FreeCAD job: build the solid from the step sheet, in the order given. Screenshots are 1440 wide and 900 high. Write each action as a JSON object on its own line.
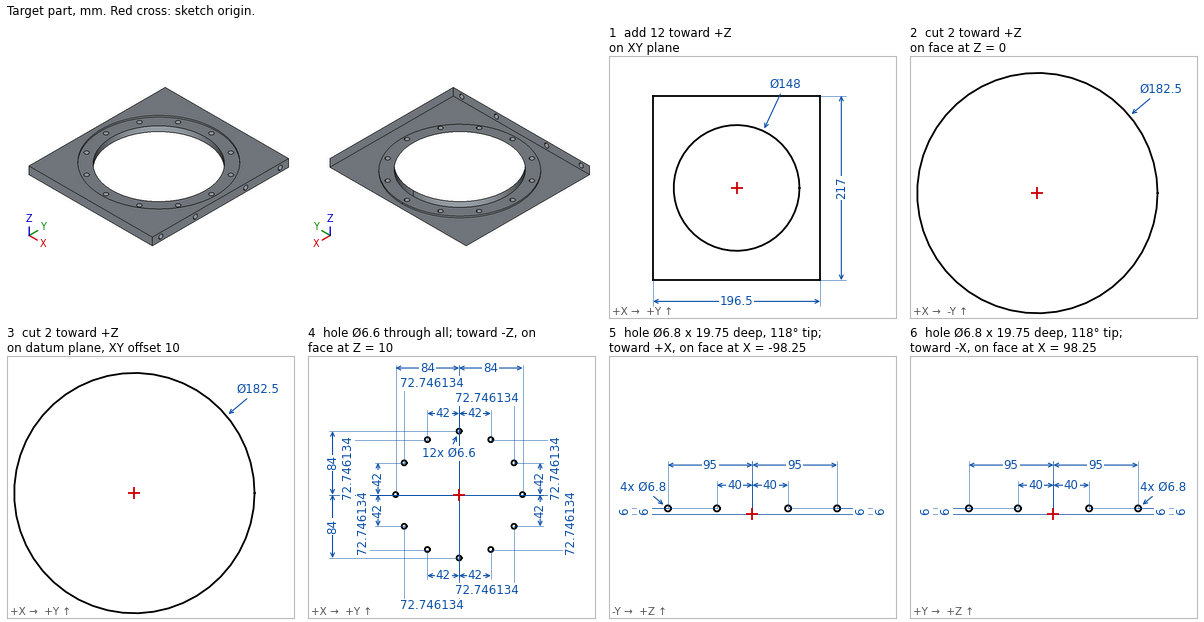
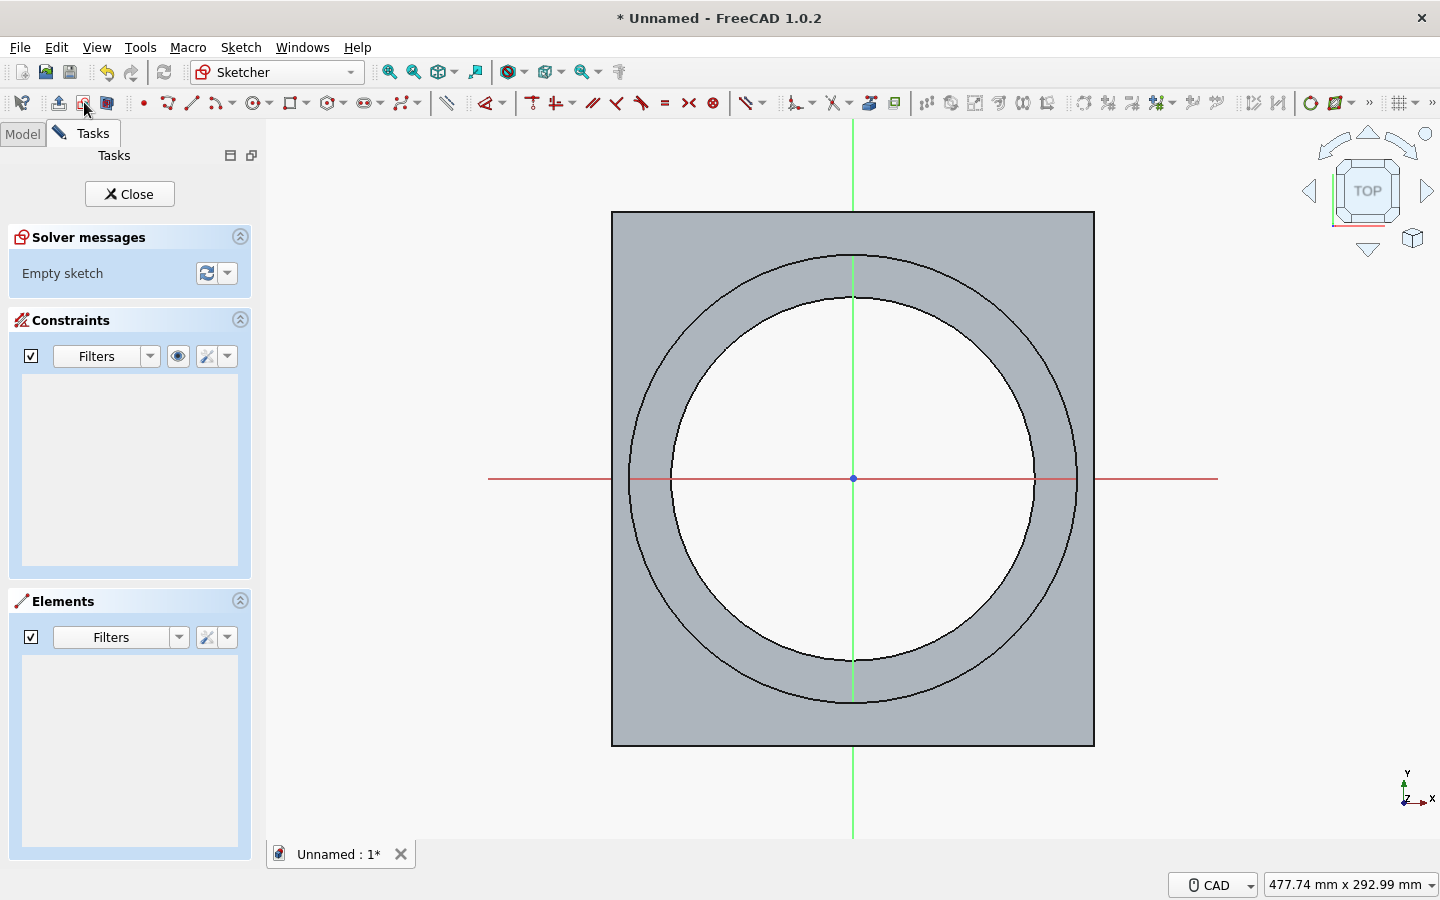
{"action": "left_click", "coordinate": [254, 104]}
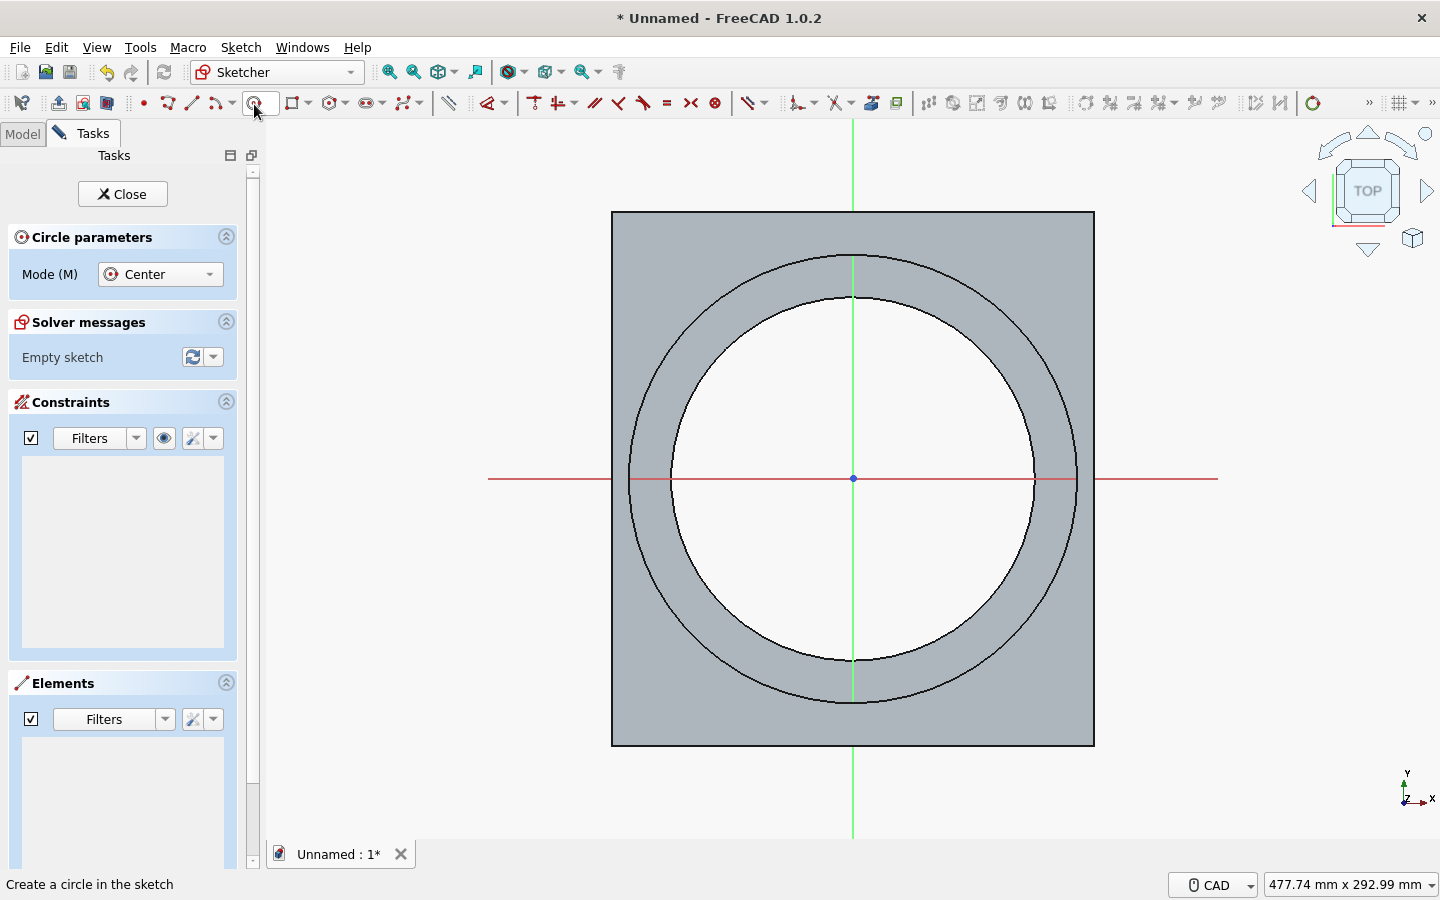
{"action": "scroll", "coordinate": [853, 273], "scroll_direction": "up", "scroll_amount": 6}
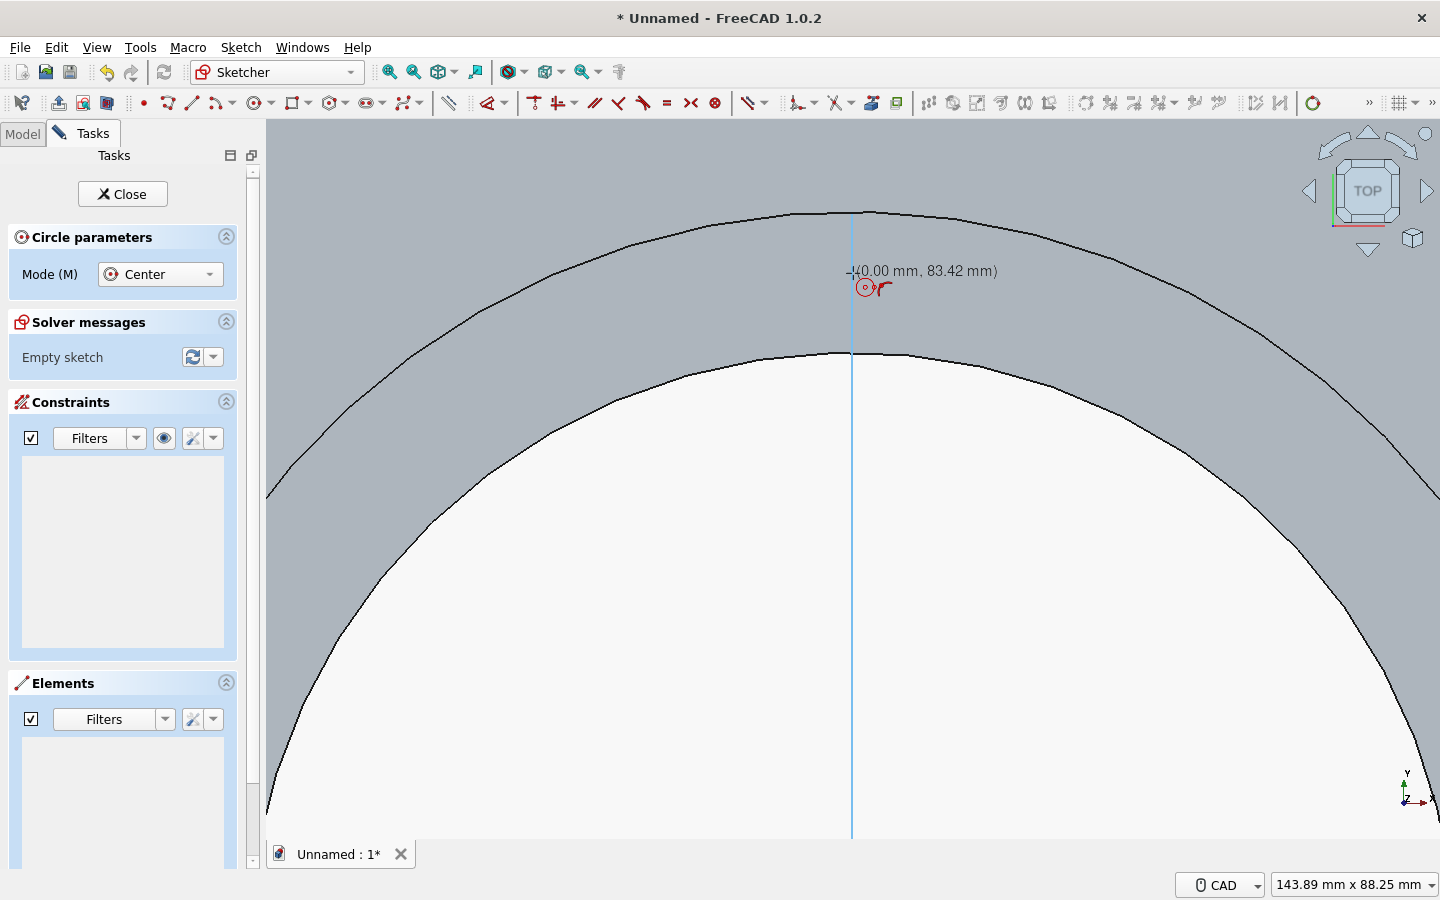
{"action": "left_click", "coordinate": [852, 271]}
{"action": "mouse_move", "coordinate": [871, 252]}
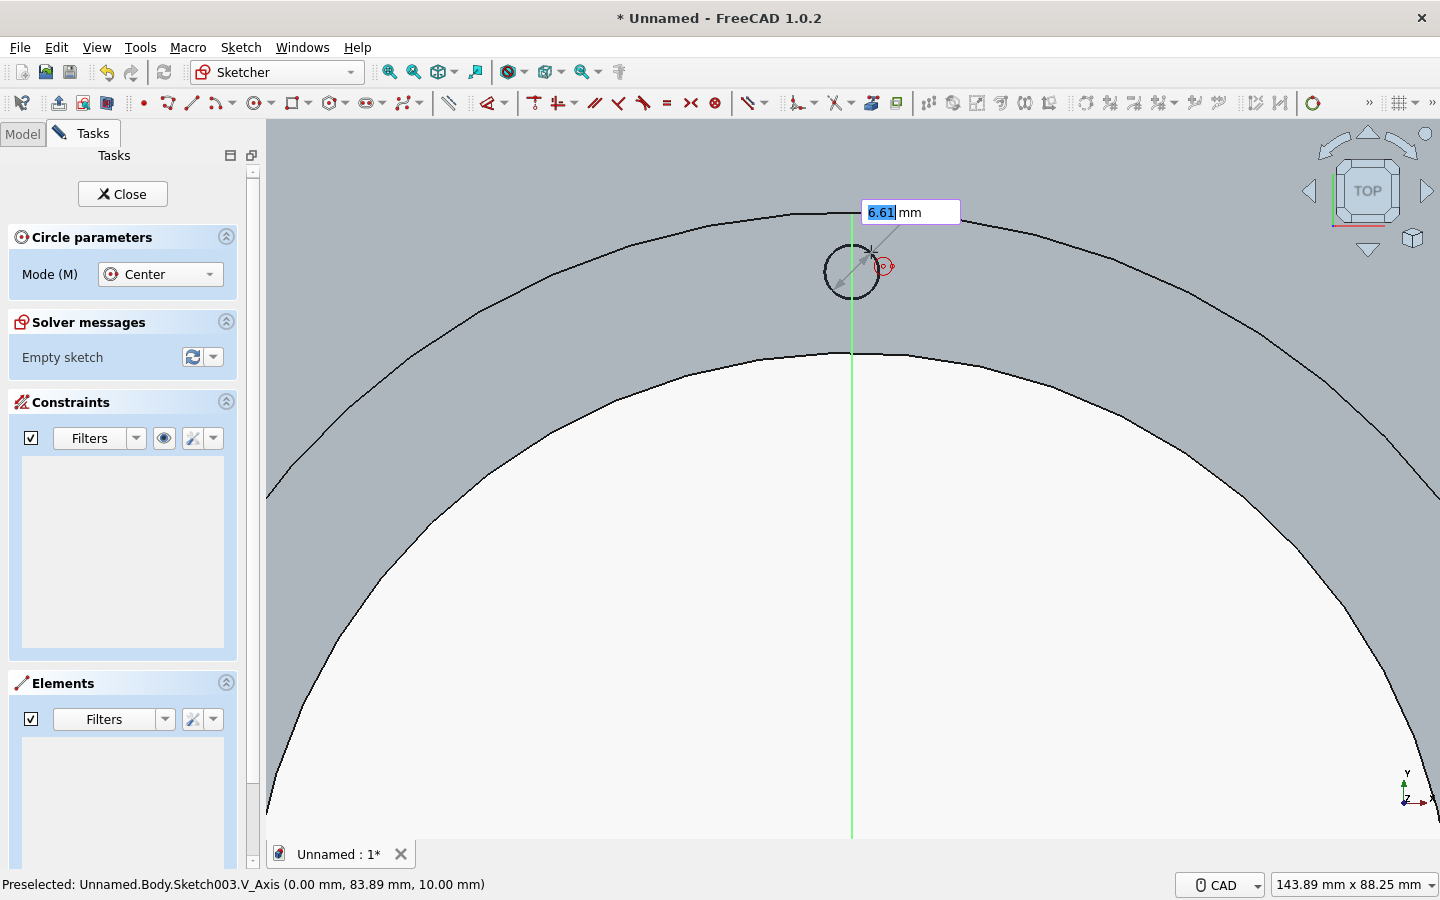
{"action": "type", "text": "6.6"}
{"action": "key", "text": "Return"}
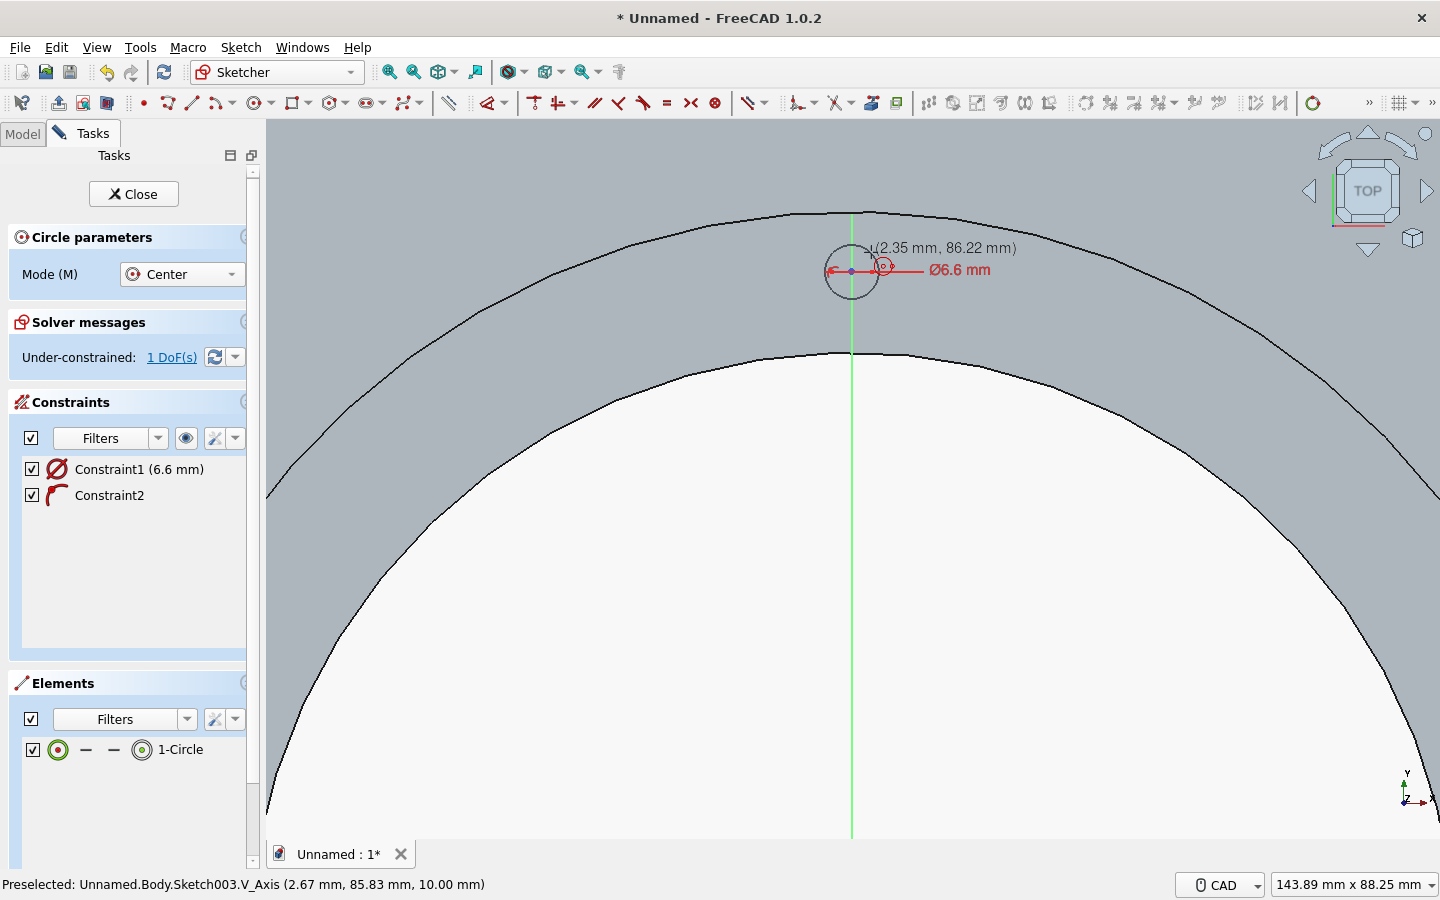
{"action": "left_click", "coordinate": [1195, 363]}
{"action": "mouse_move", "coordinate": [1214, 344]}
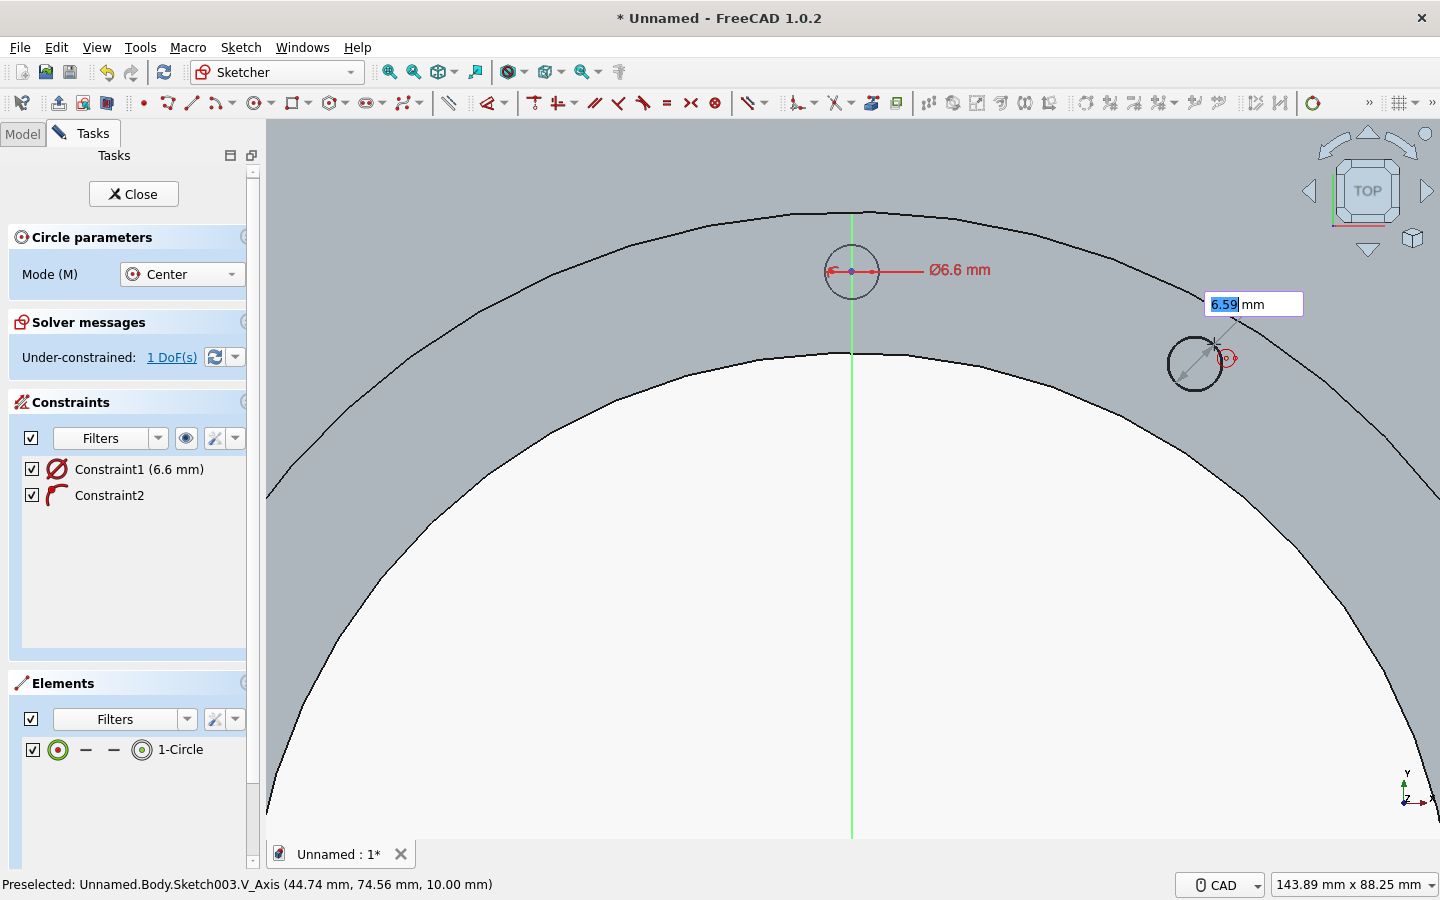
{"action": "type", "text": "6.6"}
{"action": "key", "text": "Return"}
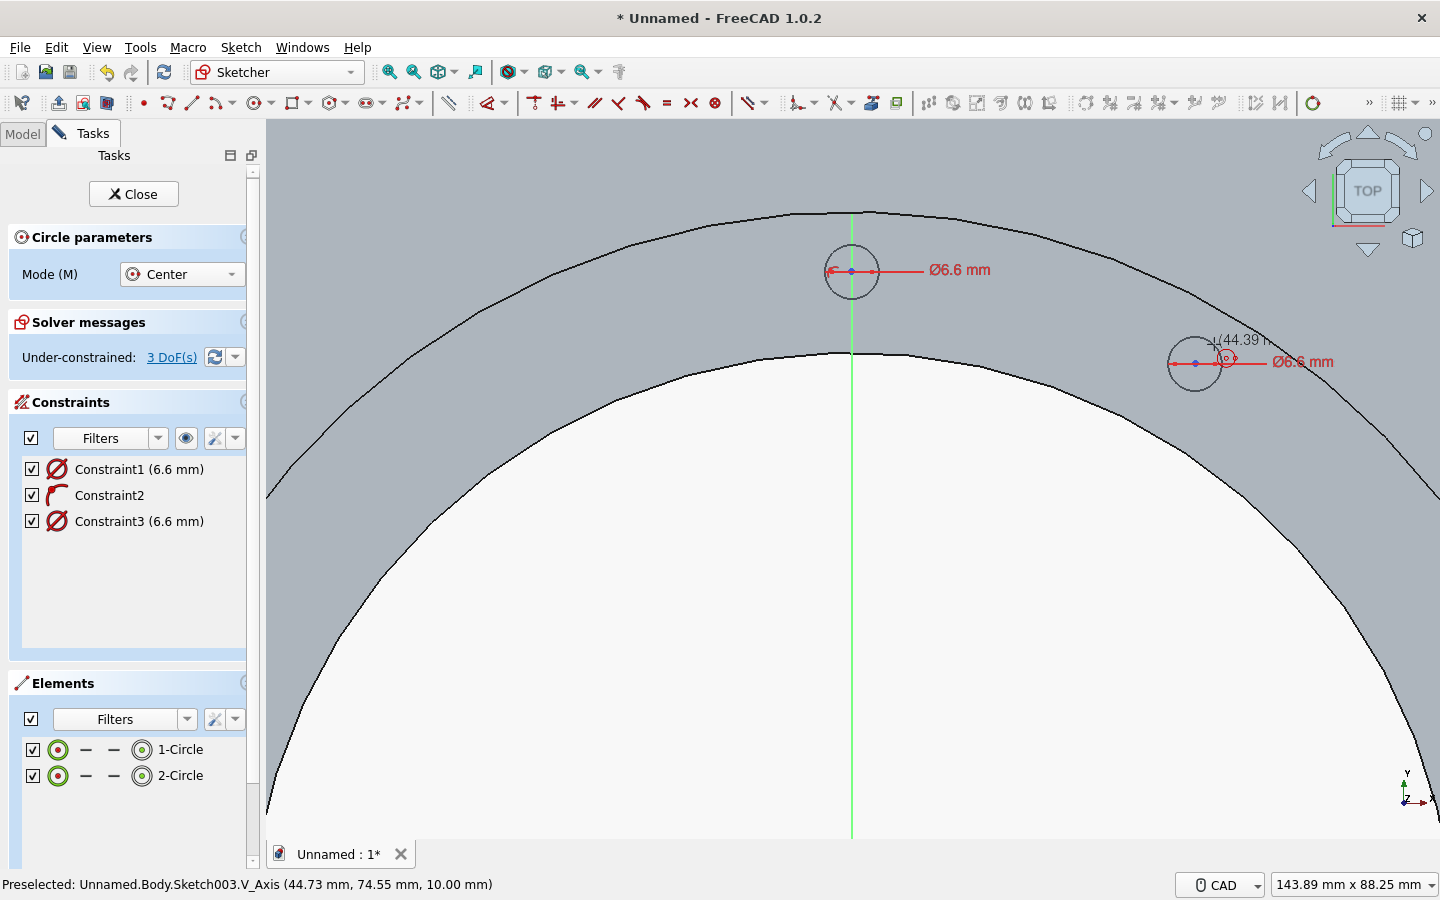
{"action": "scroll", "coordinate": [755, 273], "scroll_direction": "down", "scroll_amount": 6}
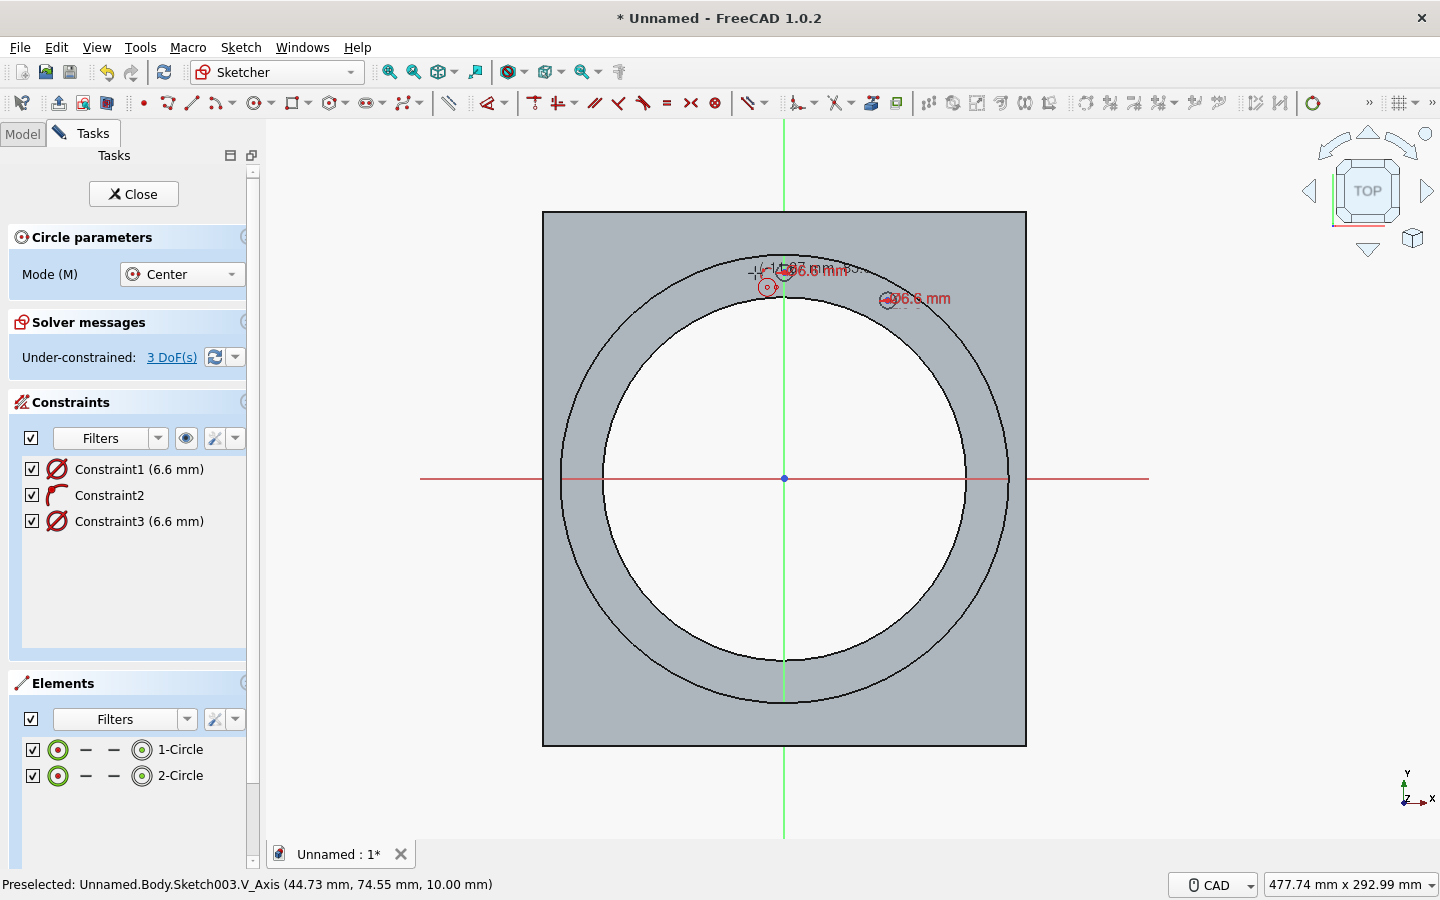
{"action": "scroll", "coordinate": [963, 376], "scroll_direction": "up", "scroll_amount": 6}